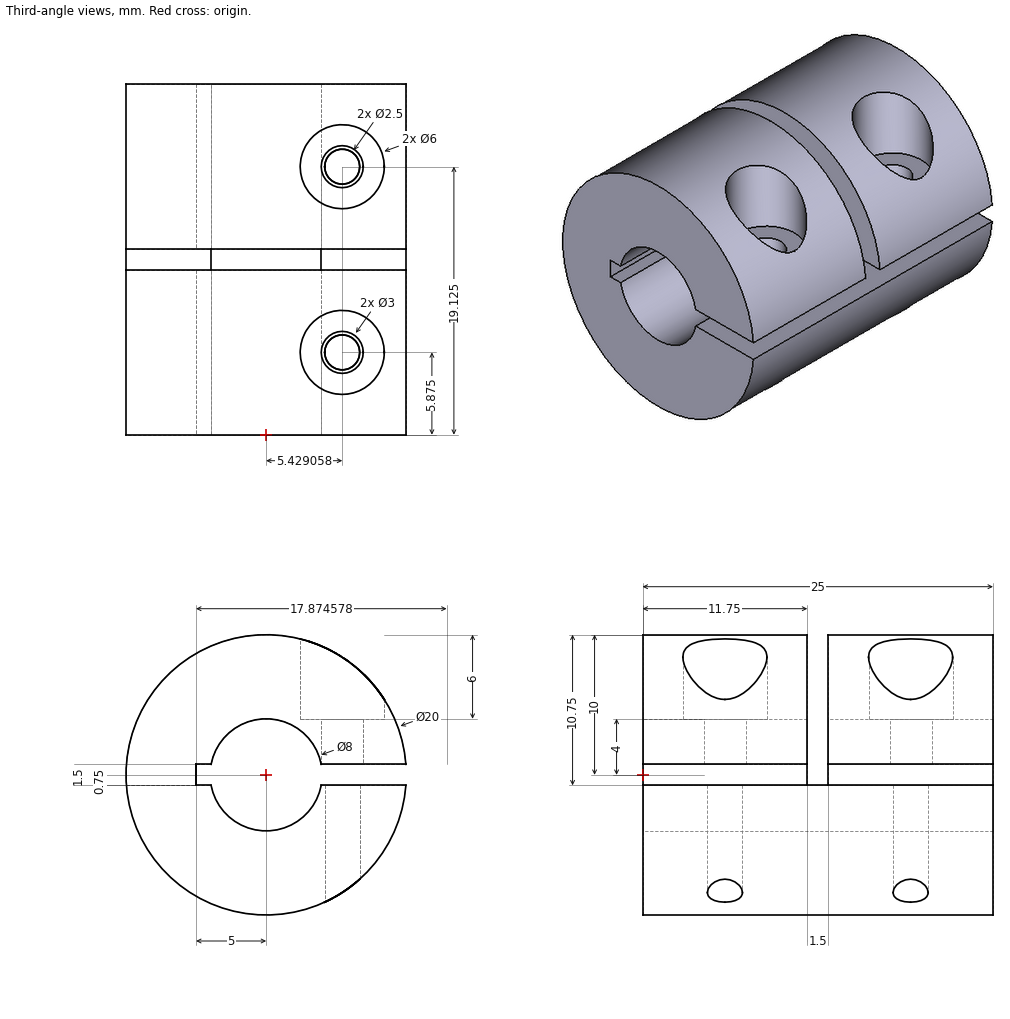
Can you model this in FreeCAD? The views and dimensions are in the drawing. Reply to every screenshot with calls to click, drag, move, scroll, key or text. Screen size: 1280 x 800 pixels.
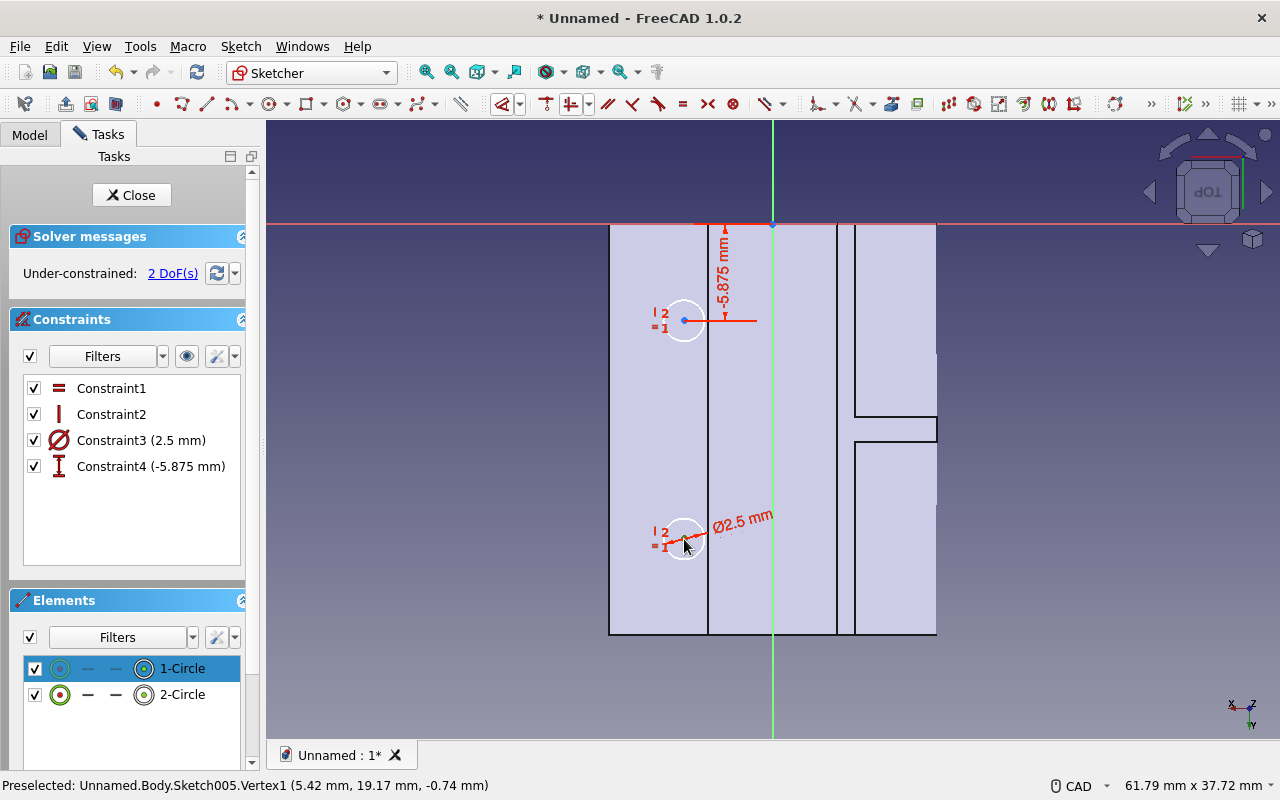
click(520, 104)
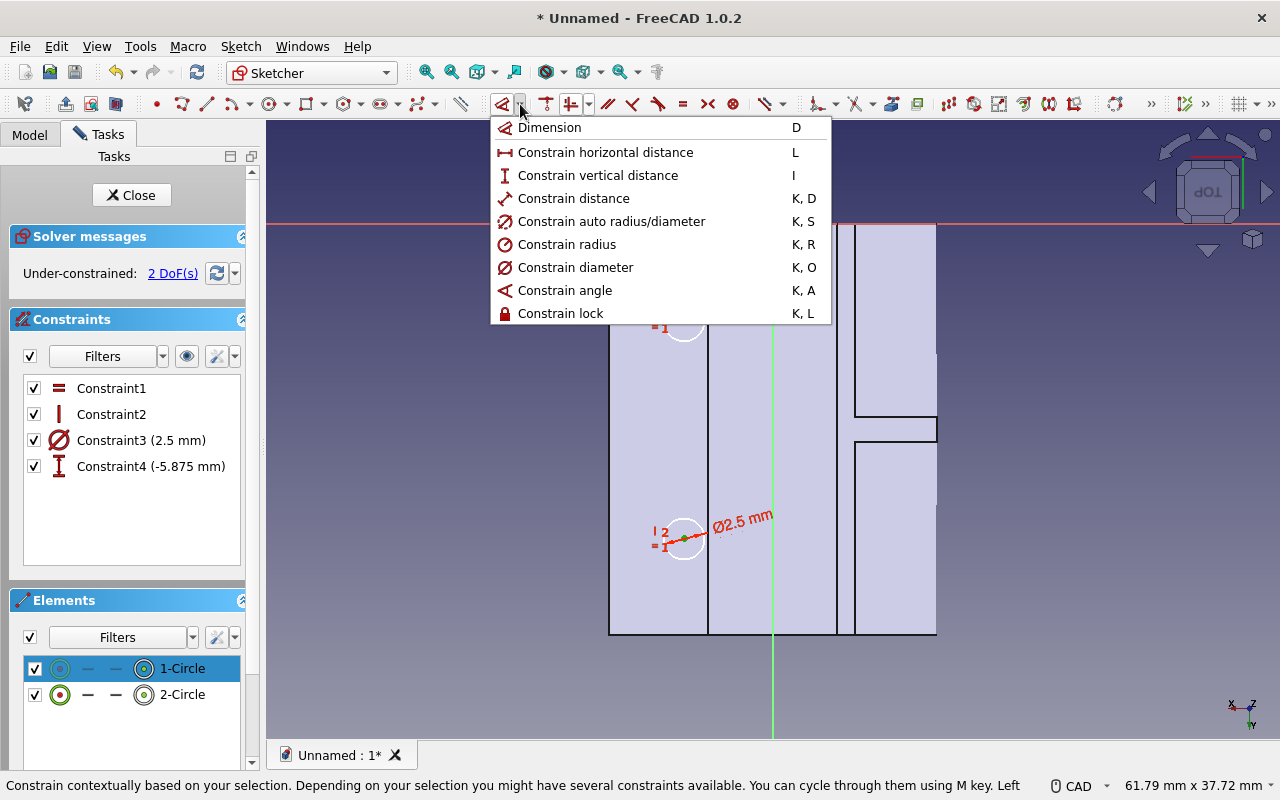
click(661, 176)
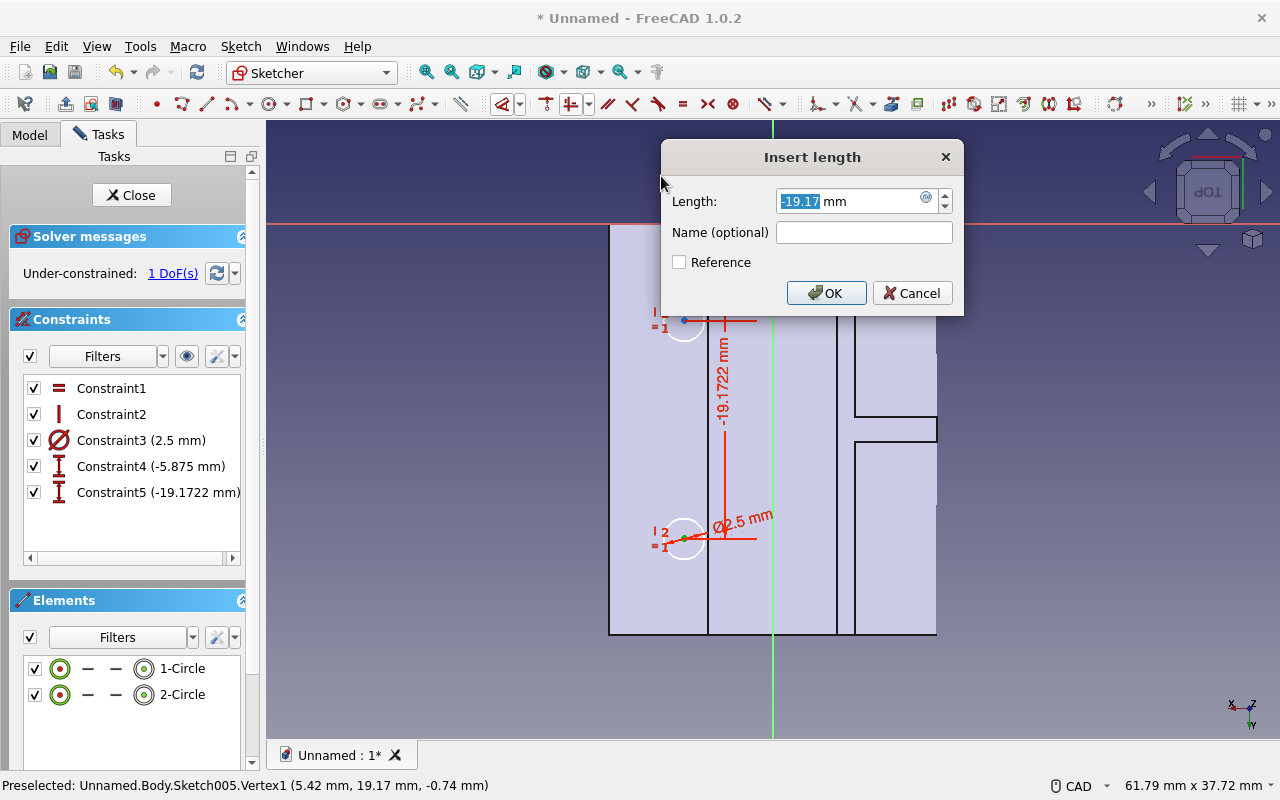
text(-19.125)
key(Return)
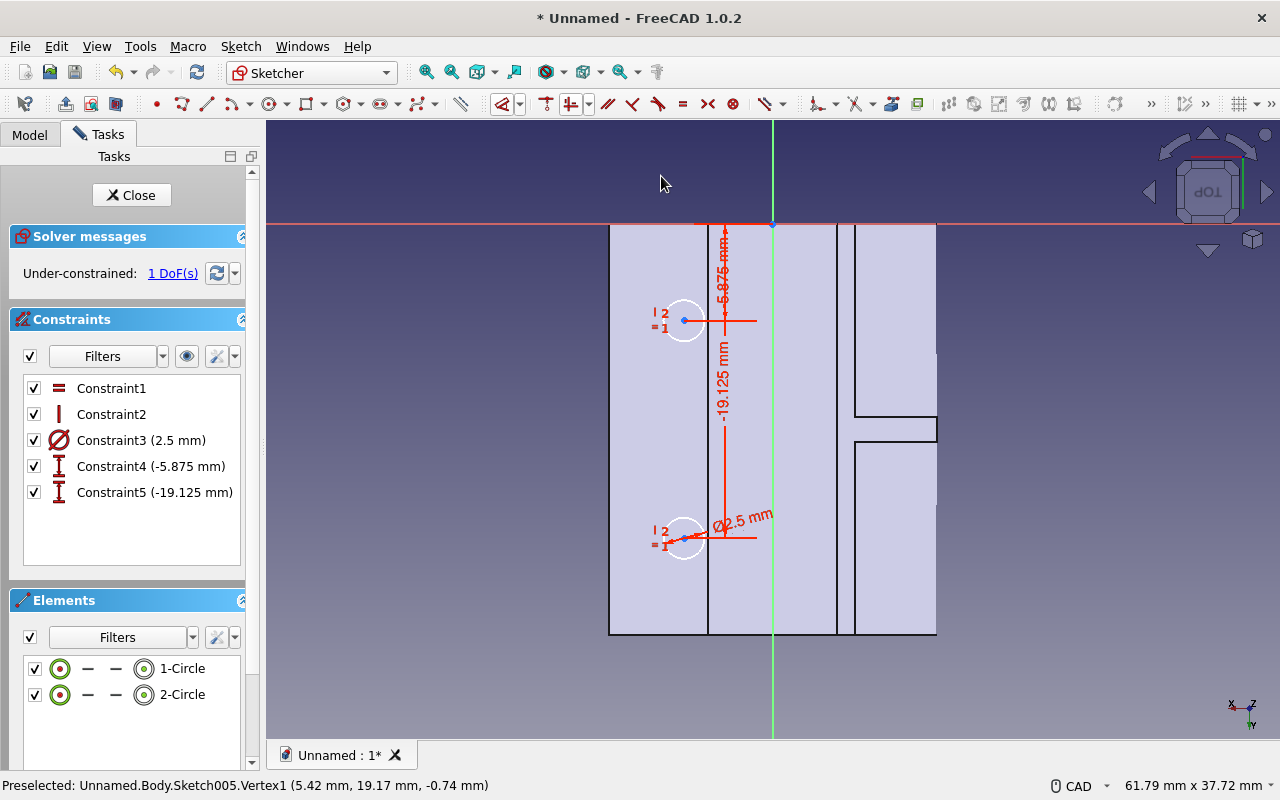
click(684, 538)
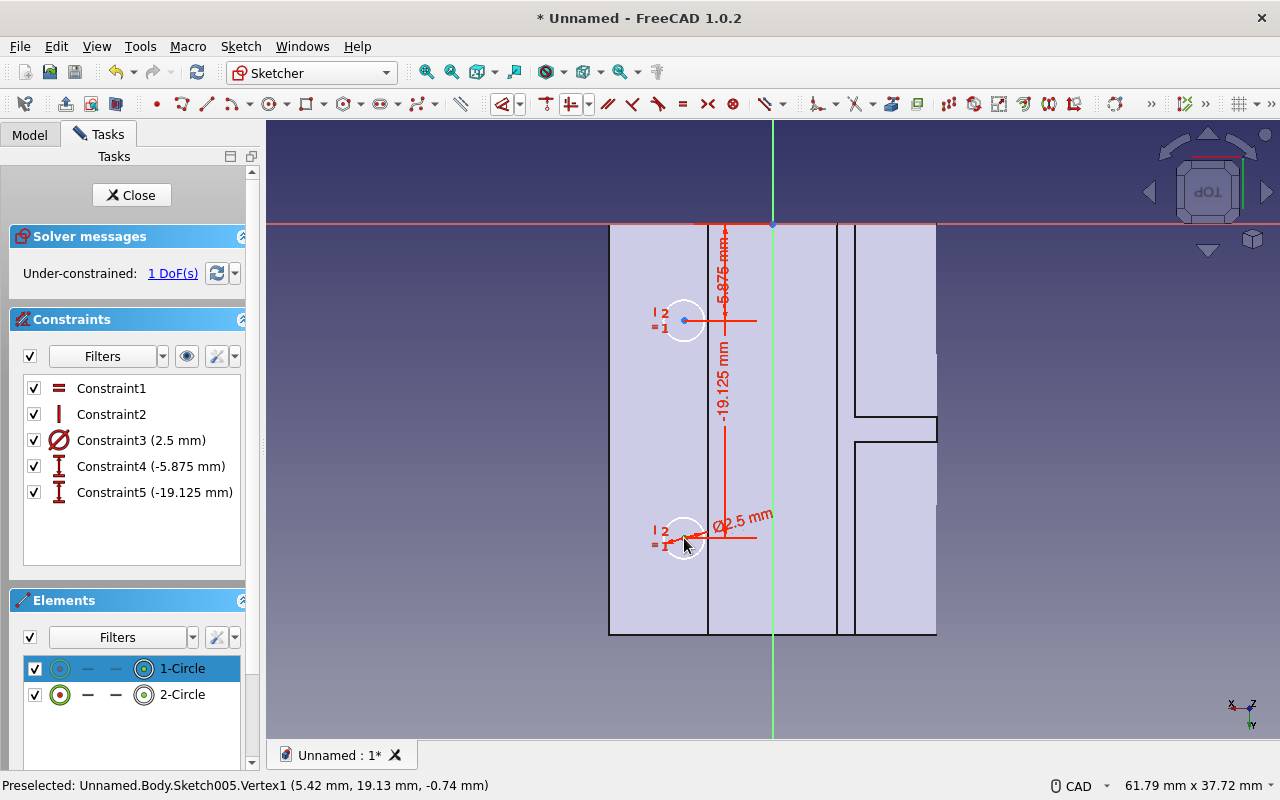
key(l)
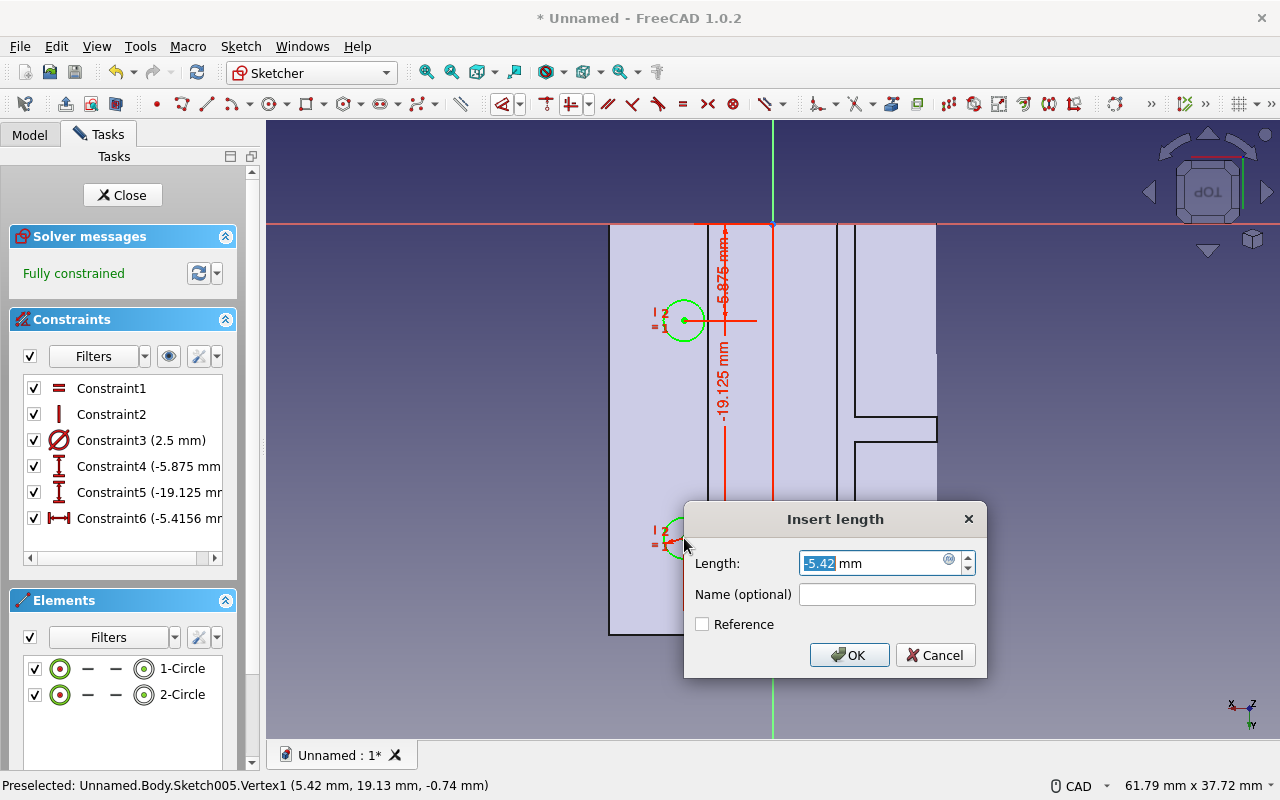
text(-5.429058)
key(Return)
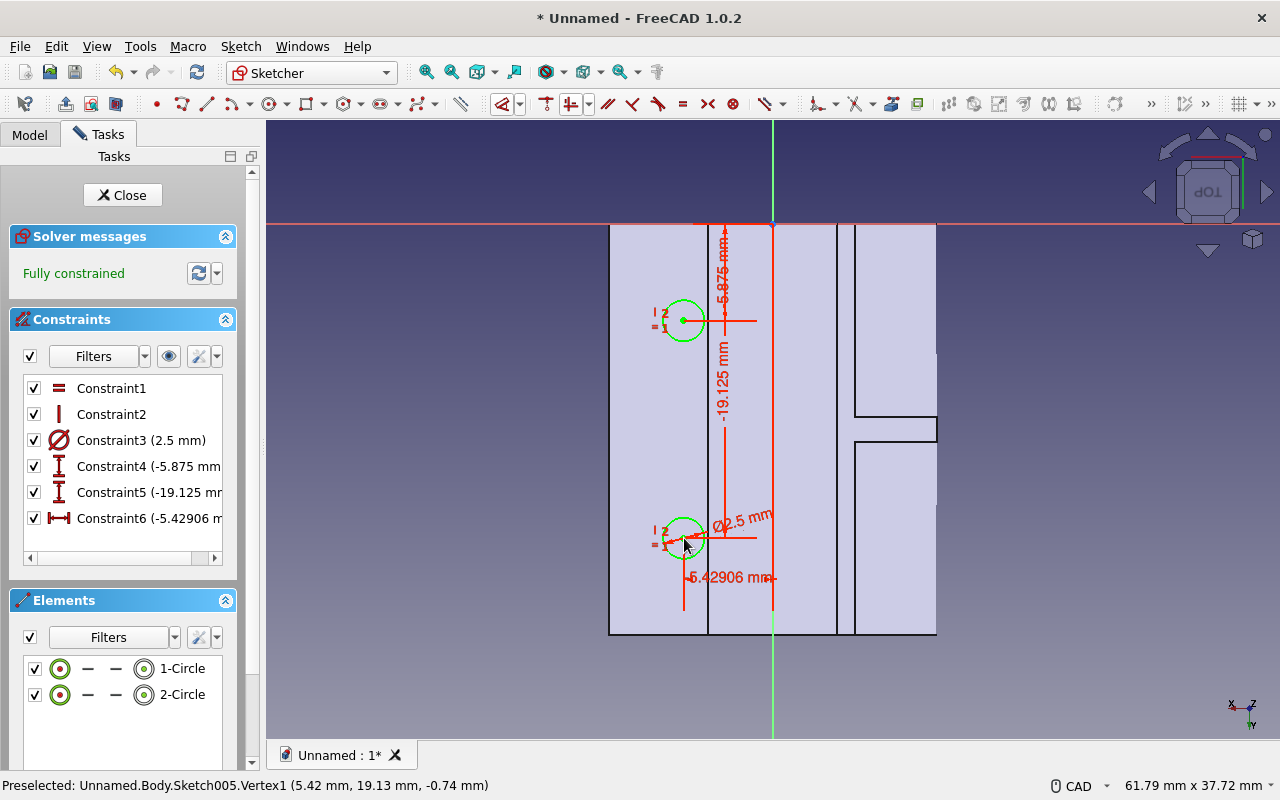
click(123, 195)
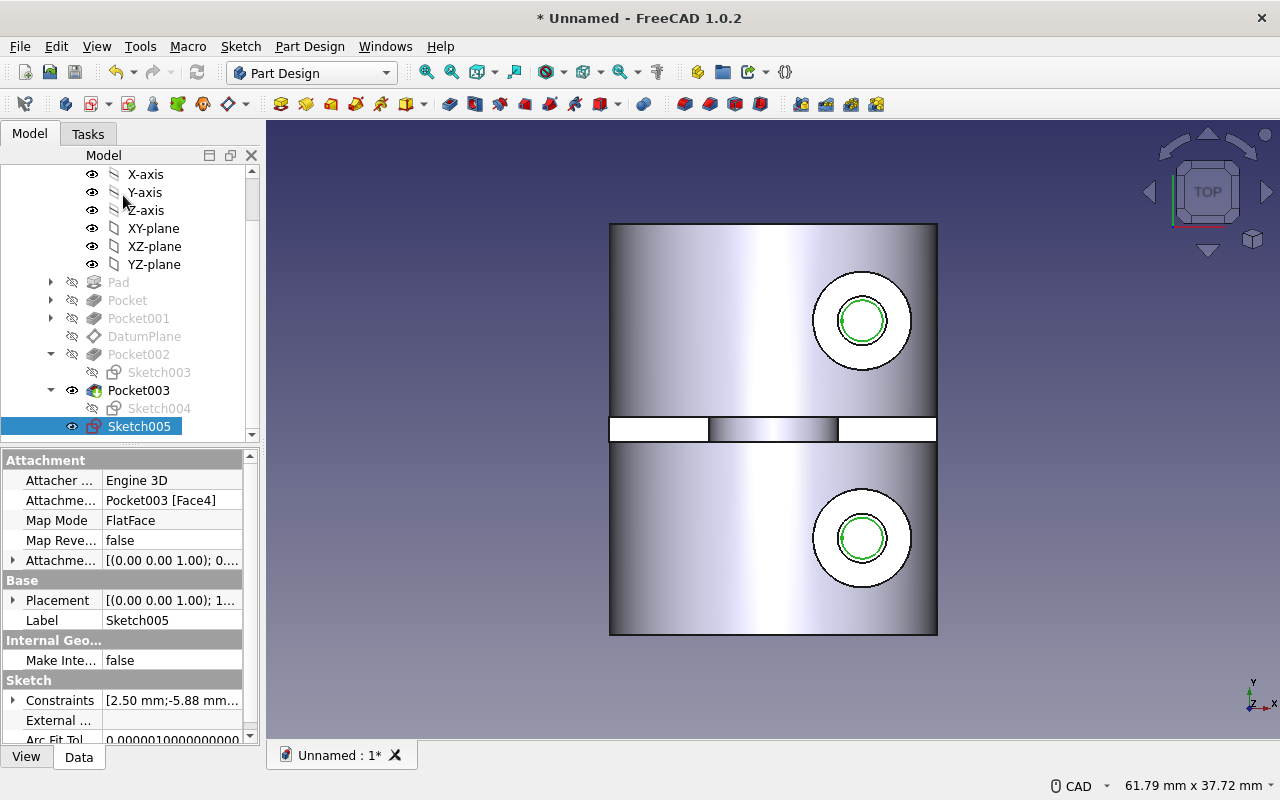
click(450, 104)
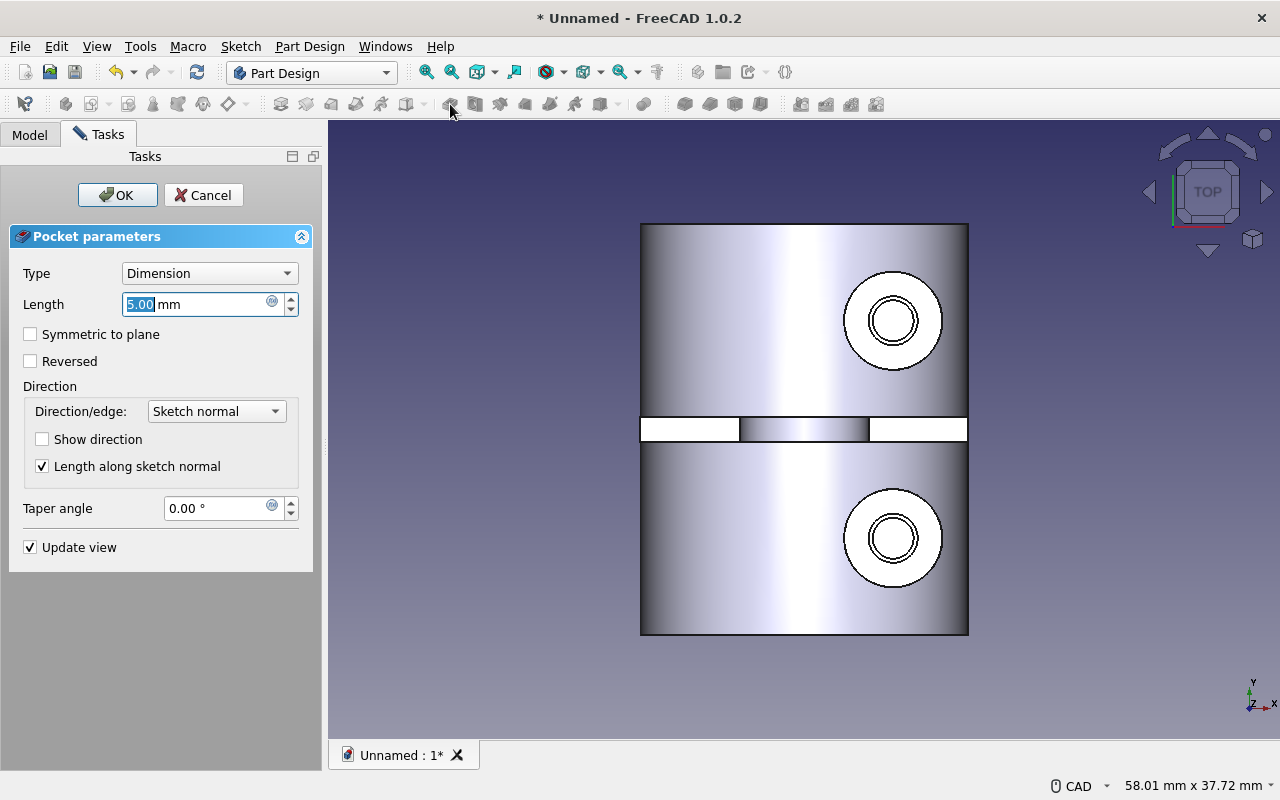
click(210, 274)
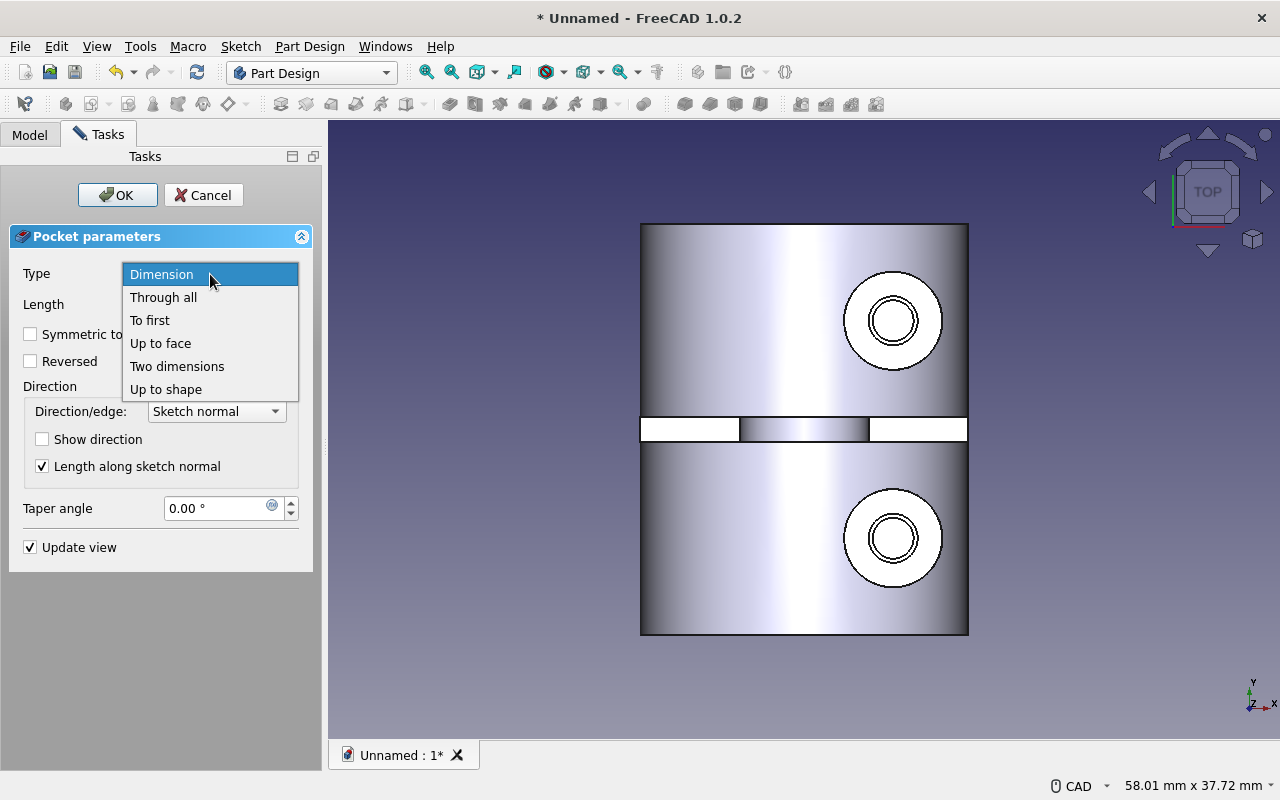
click(208, 298)